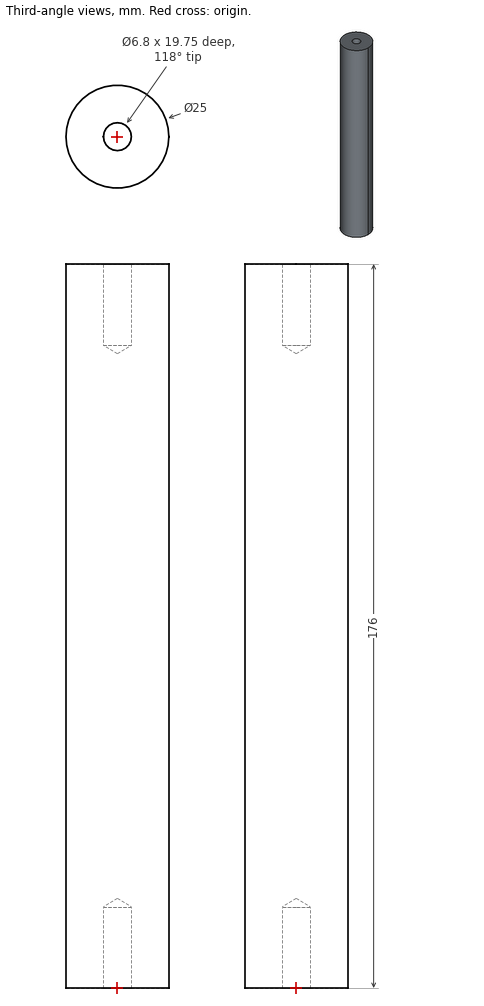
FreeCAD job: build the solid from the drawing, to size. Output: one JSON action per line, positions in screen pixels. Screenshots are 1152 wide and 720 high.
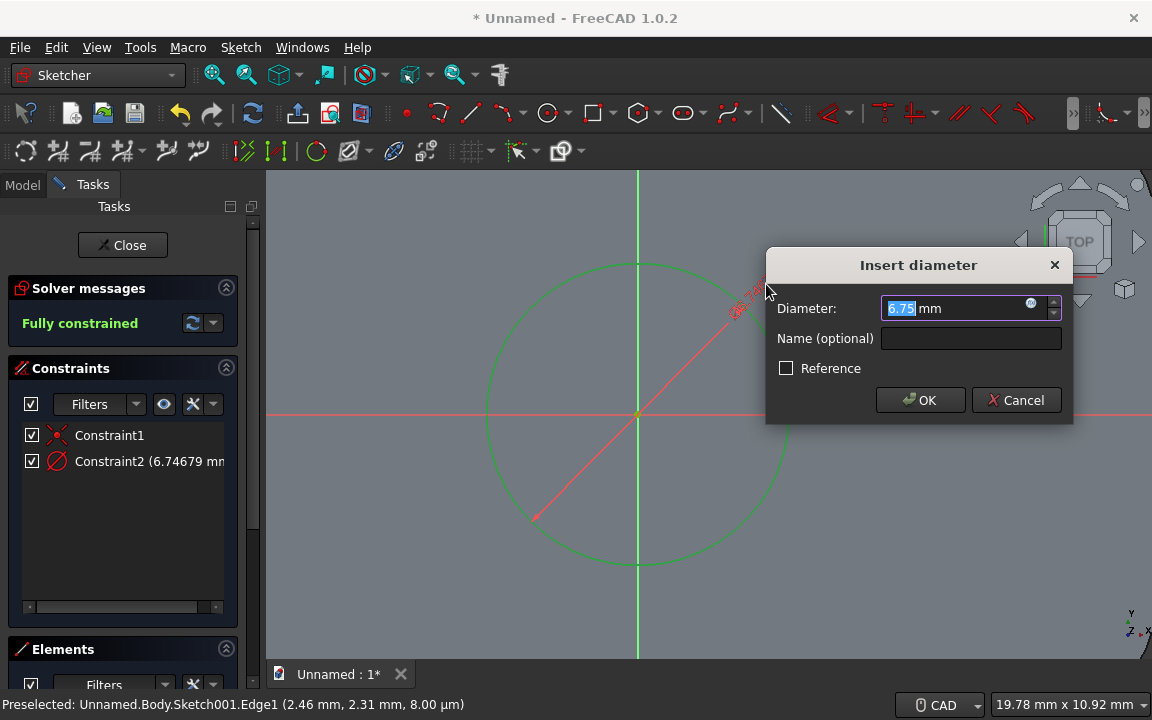
{"action": "type", "text": "6.8"}
{"action": "key", "text": "Return"}
{"action": "key", "text": "Escape"}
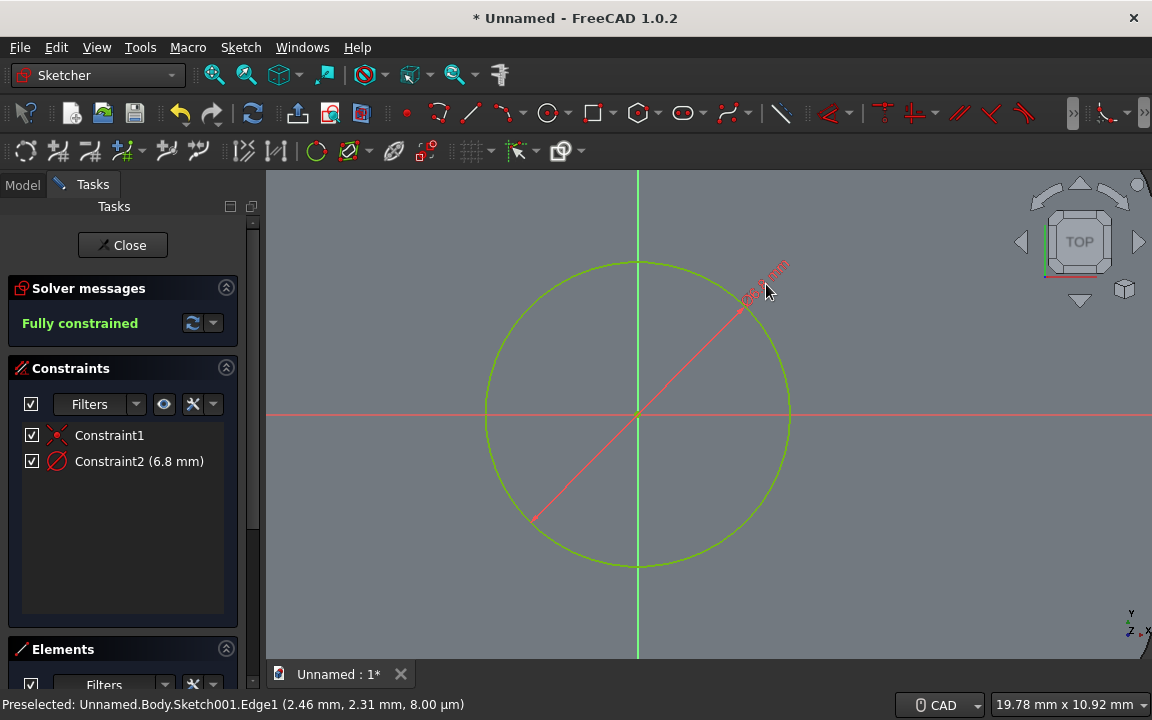
{"action": "left_click", "coordinate": [123, 245]}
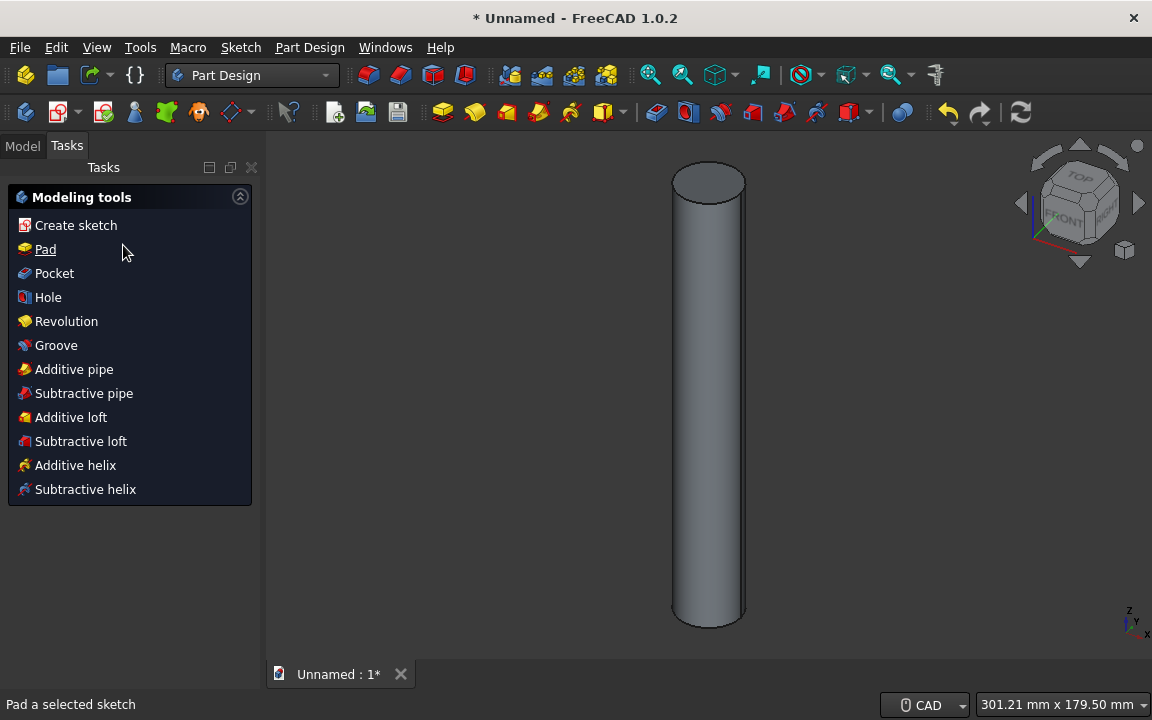
{"action": "left_click", "coordinate": [690, 112]}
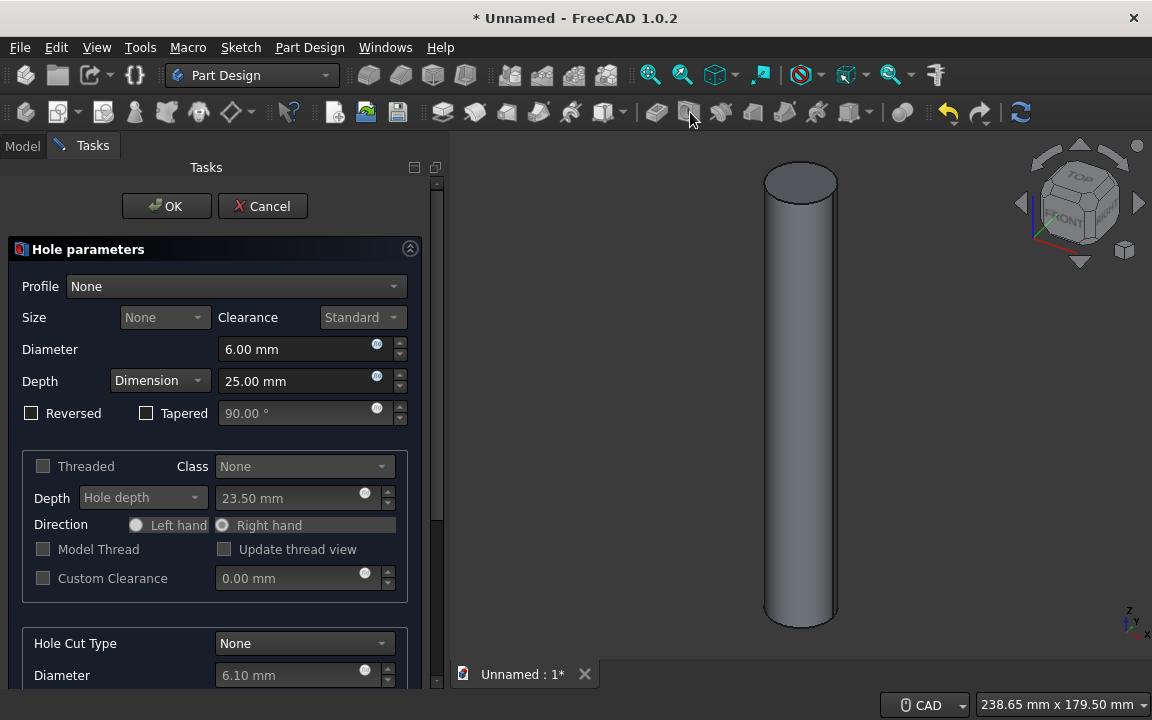
{"action": "triple_click", "coordinate": [305, 349]}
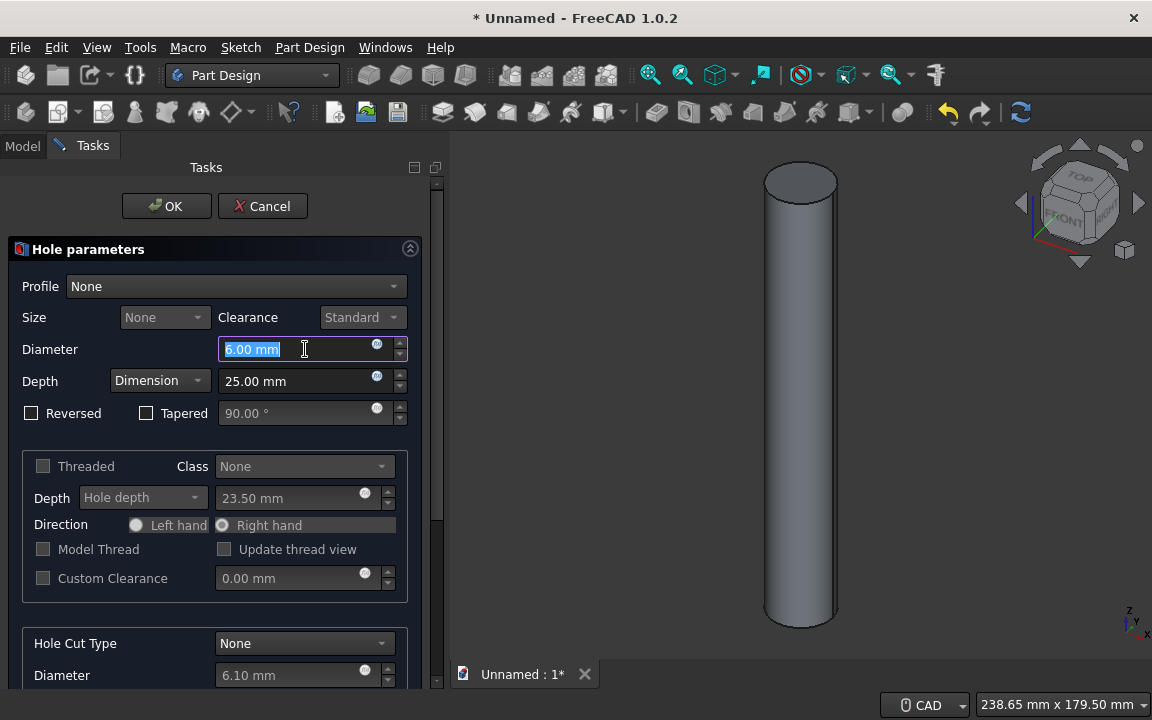
{"action": "type", "text": "6.8"}
{"action": "key", "text": "Tab"}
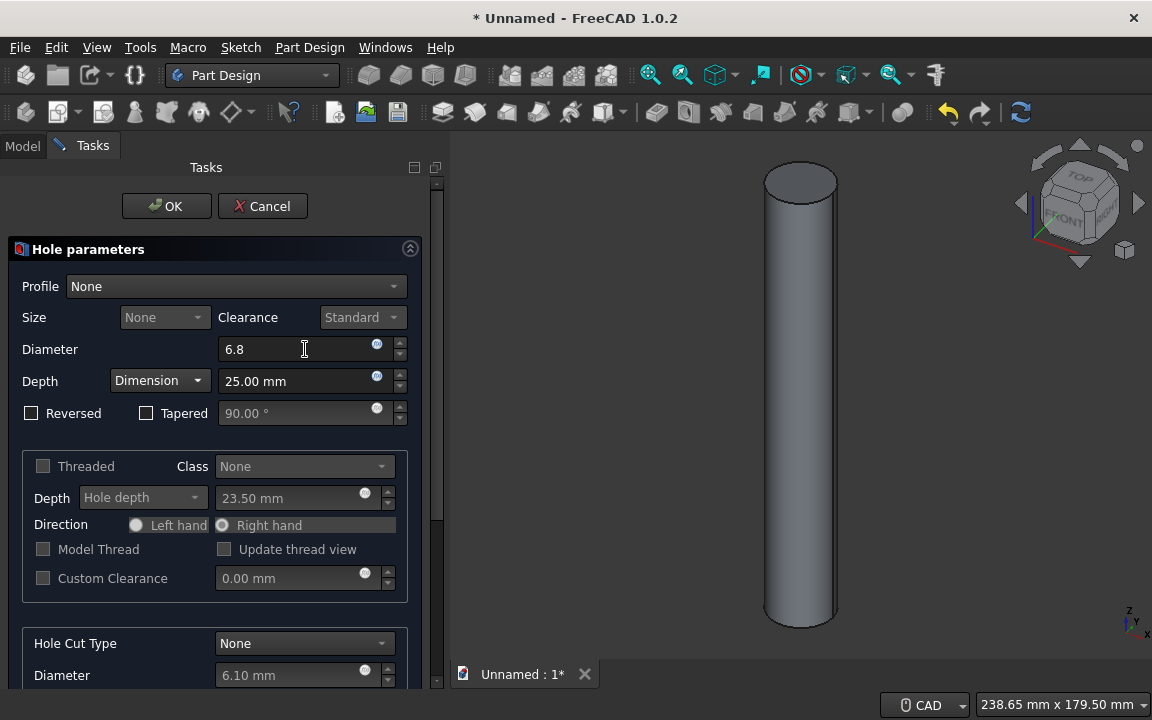
{"action": "triple_click", "coordinate": [305, 381]}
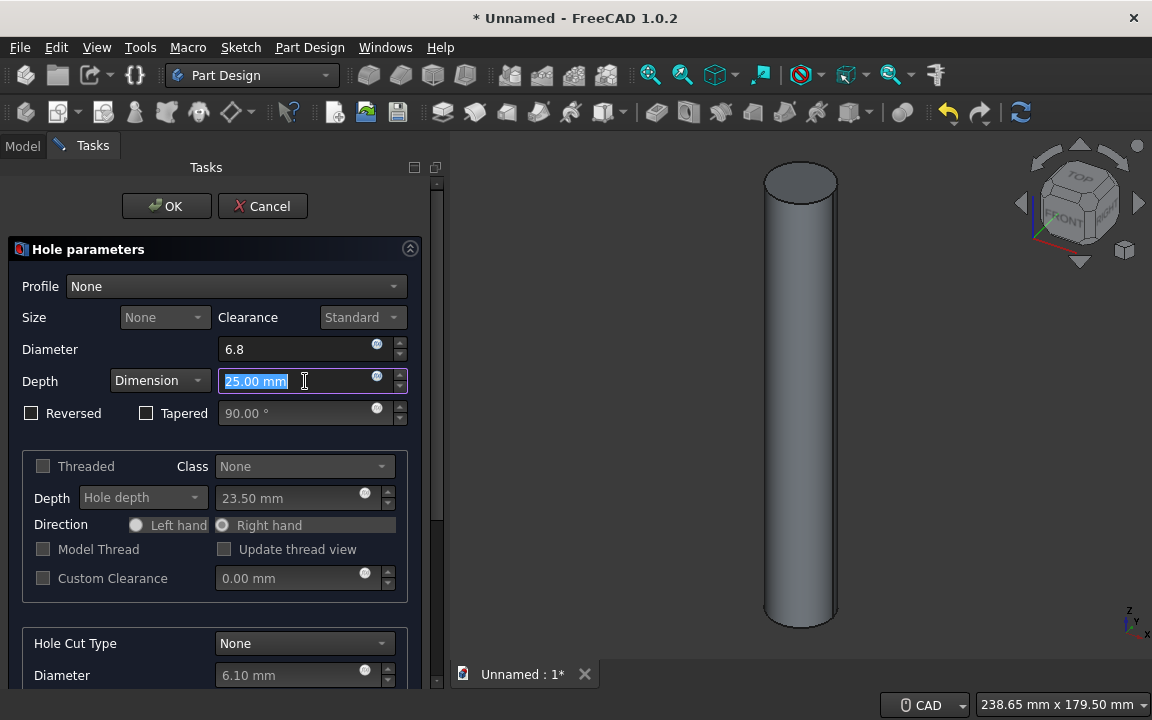
{"action": "type", "text": "19.75"}
{"action": "key", "text": "Tab"}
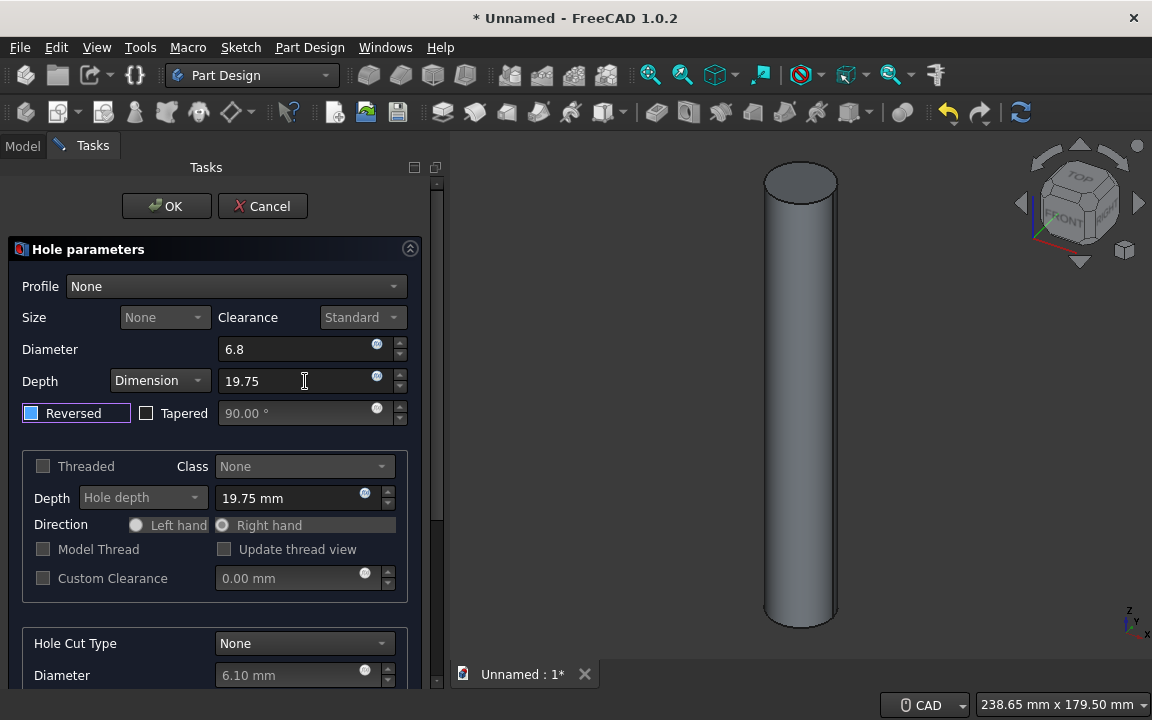
{"action": "left_click", "coordinate": [30, 413]}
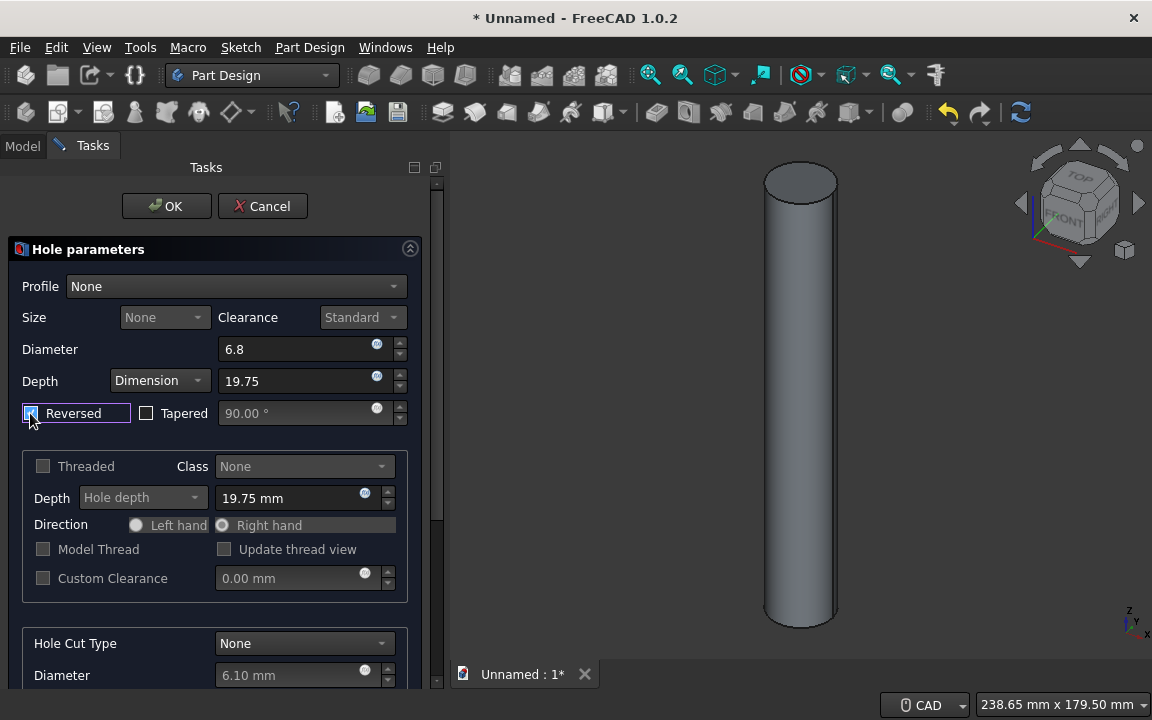
{"action": "left_click", "coordinate": [167, 206]}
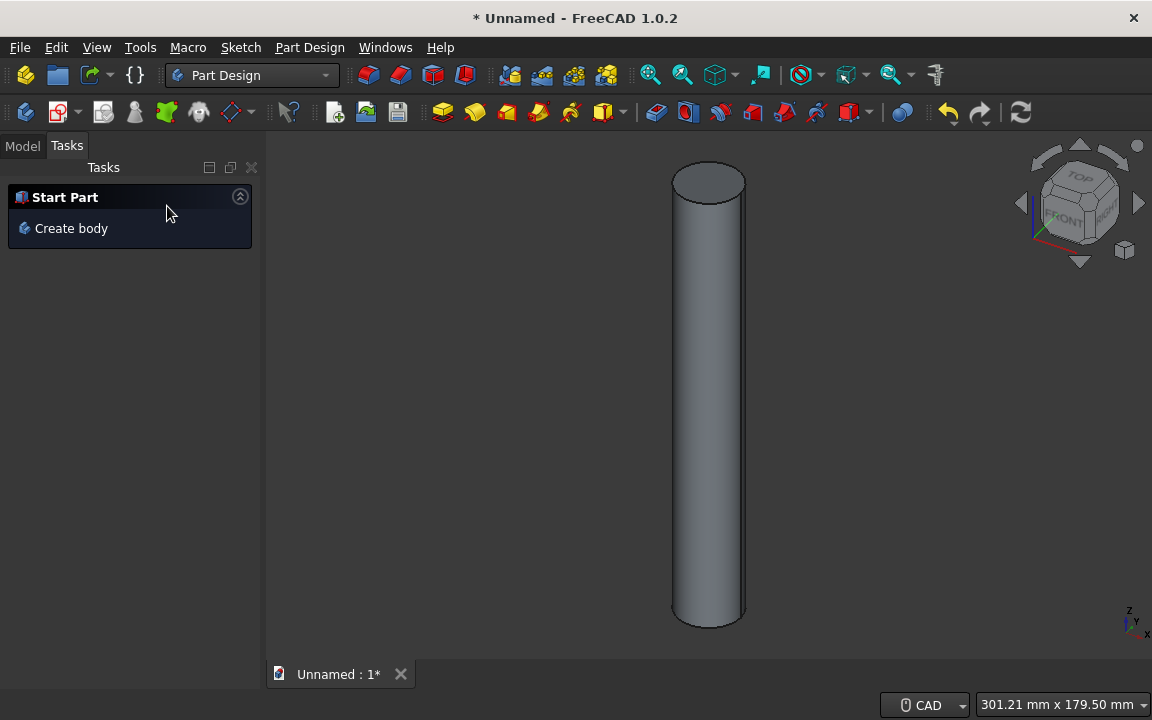
{"action": "left_click", "coordinate": [709, 182]}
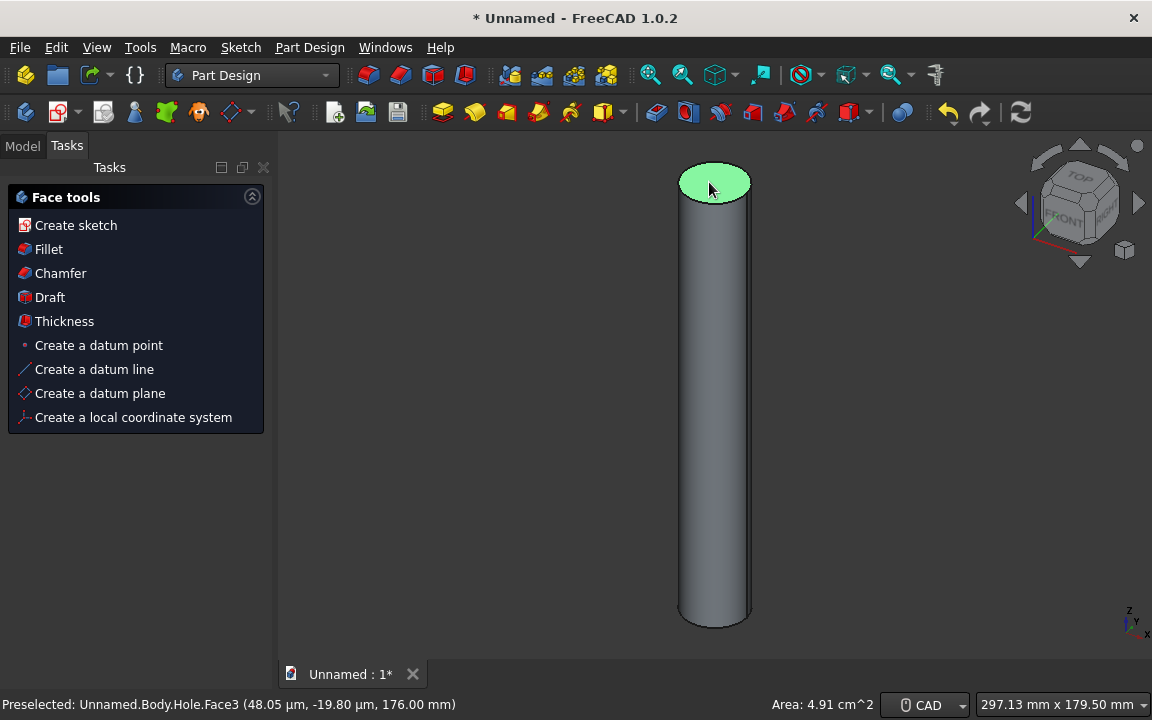
{"action": "left_click", "coordinate": [58, 112]}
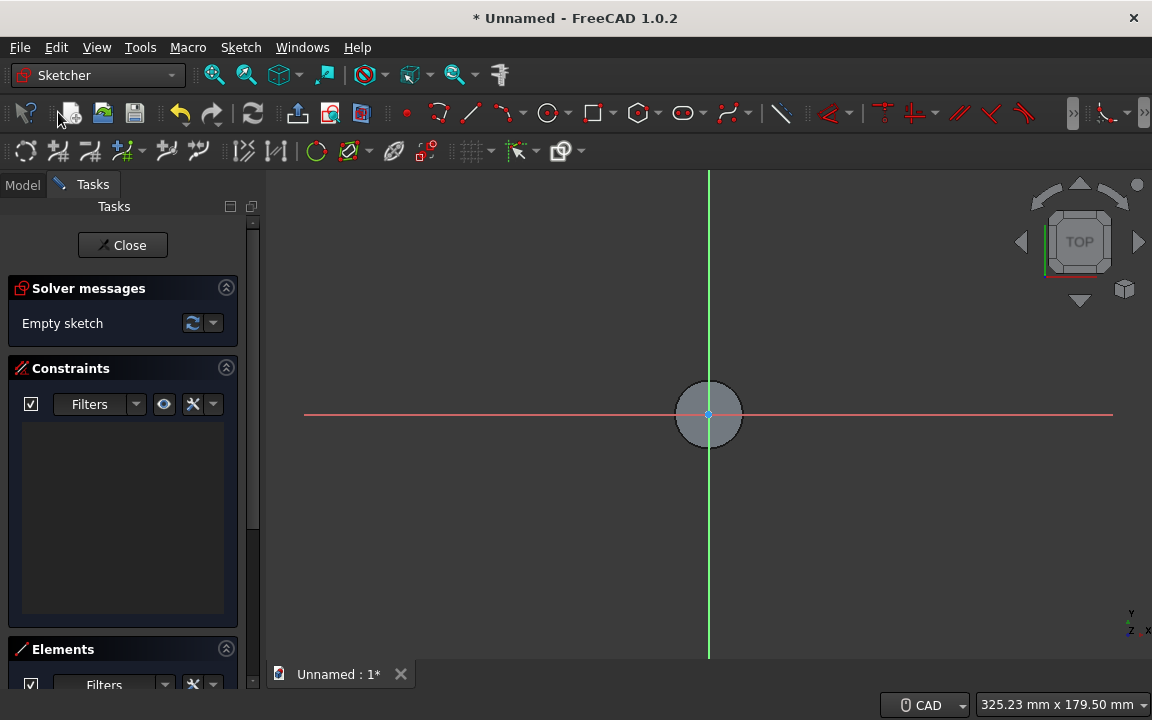
{"action": "scroll", "coordinate": [713, 415], "scroll_direction": "up", "scroll_amount": 14}